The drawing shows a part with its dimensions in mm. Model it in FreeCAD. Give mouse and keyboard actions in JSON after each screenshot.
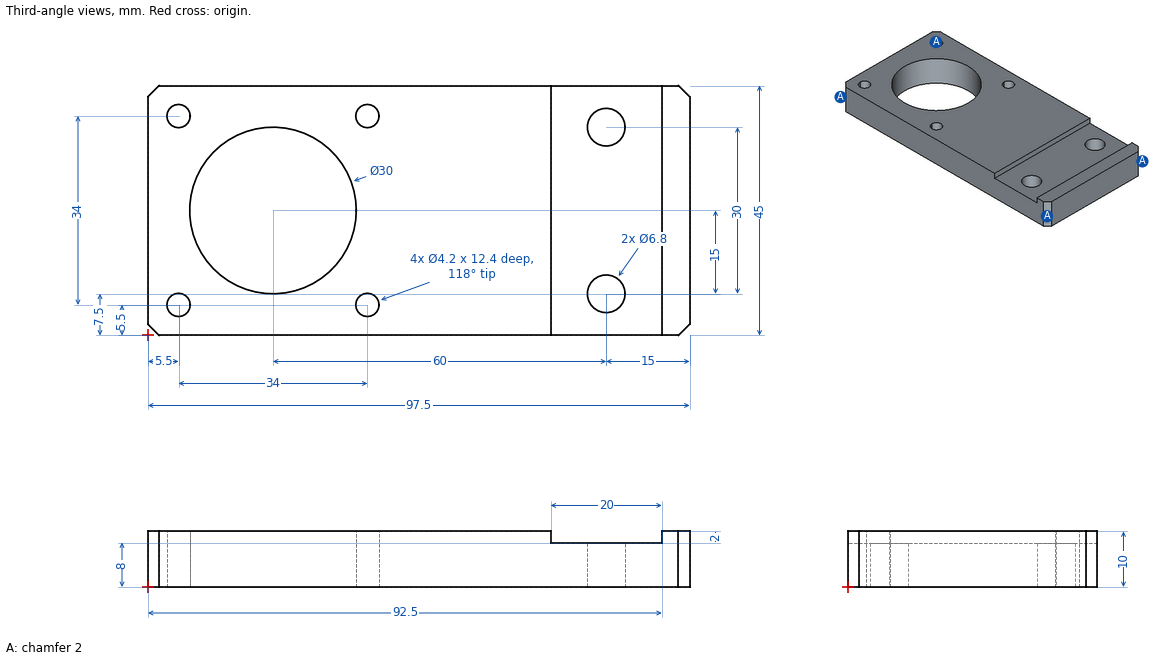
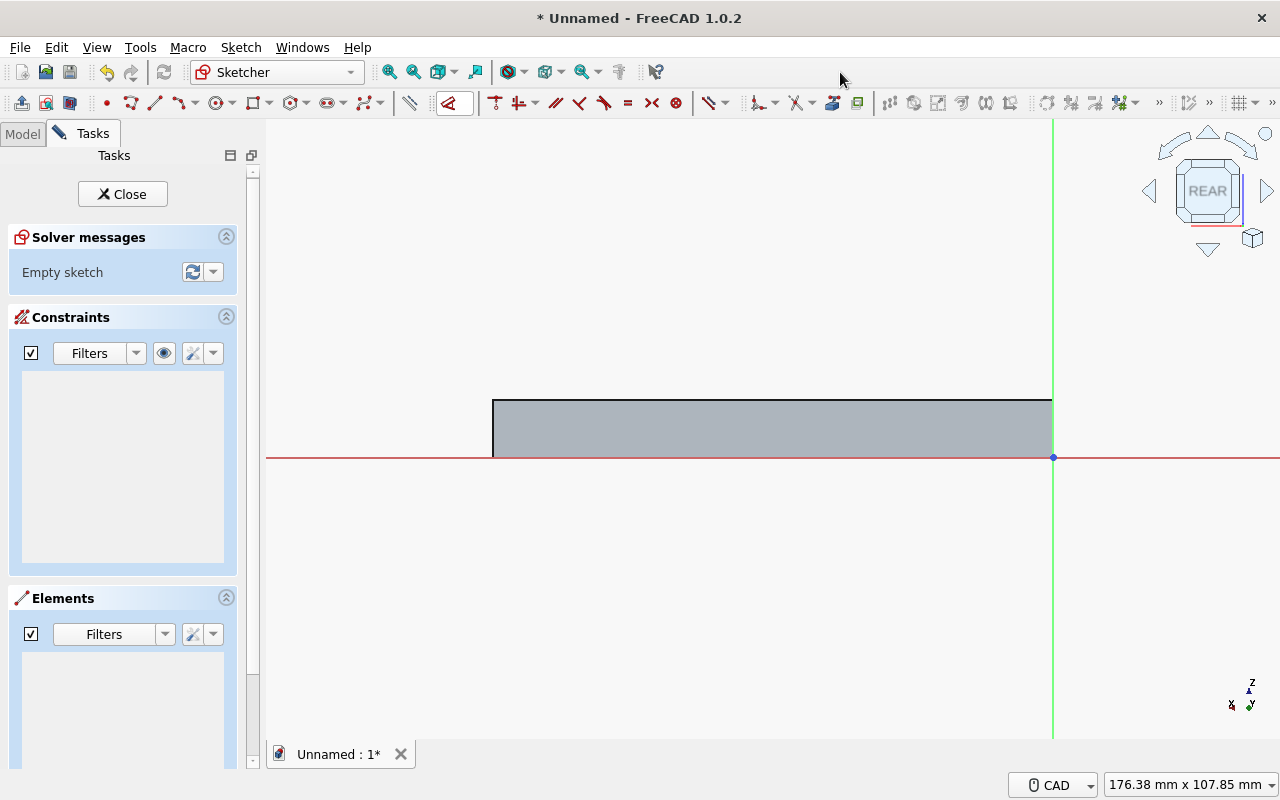
{"action": "scroll", "coordinate": [547, 400], "scroll_direction": "up", "scroll_amount": 8}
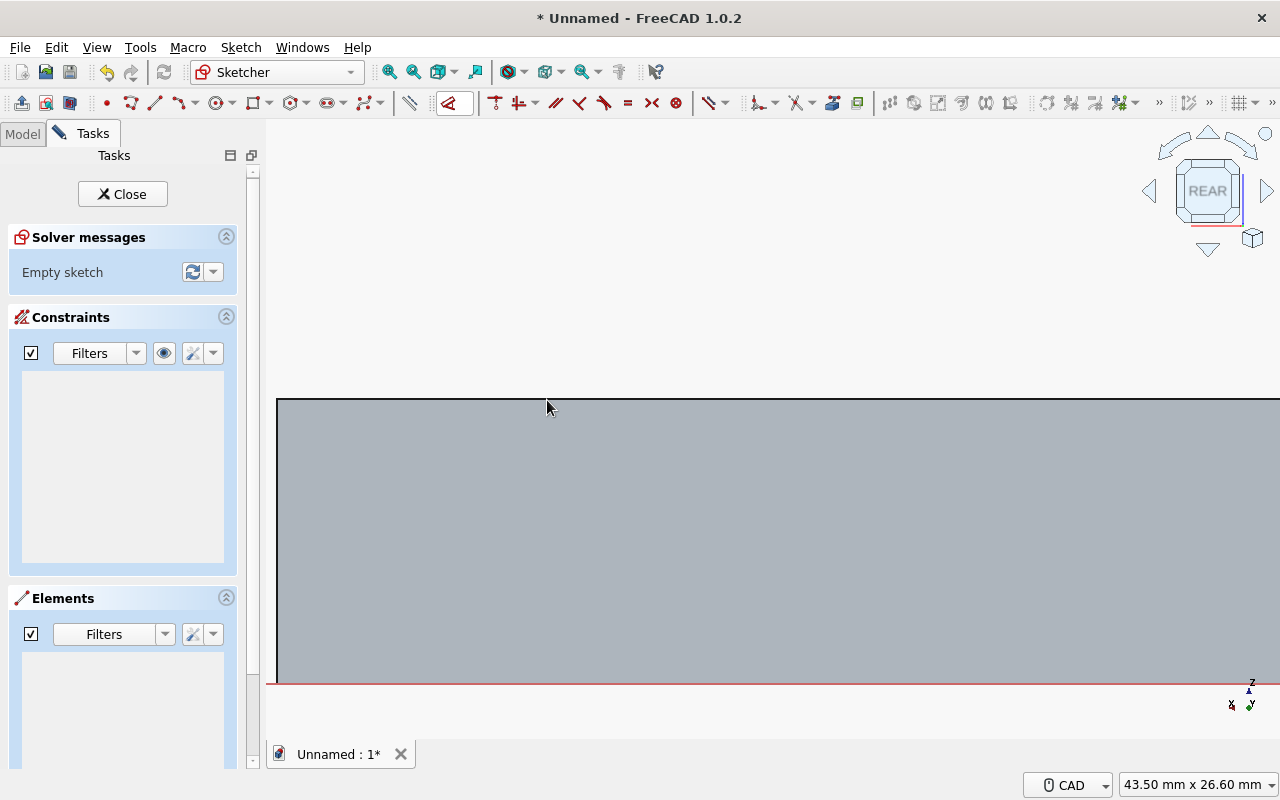
{"action": "left_click", "coordinate": [254, 104]}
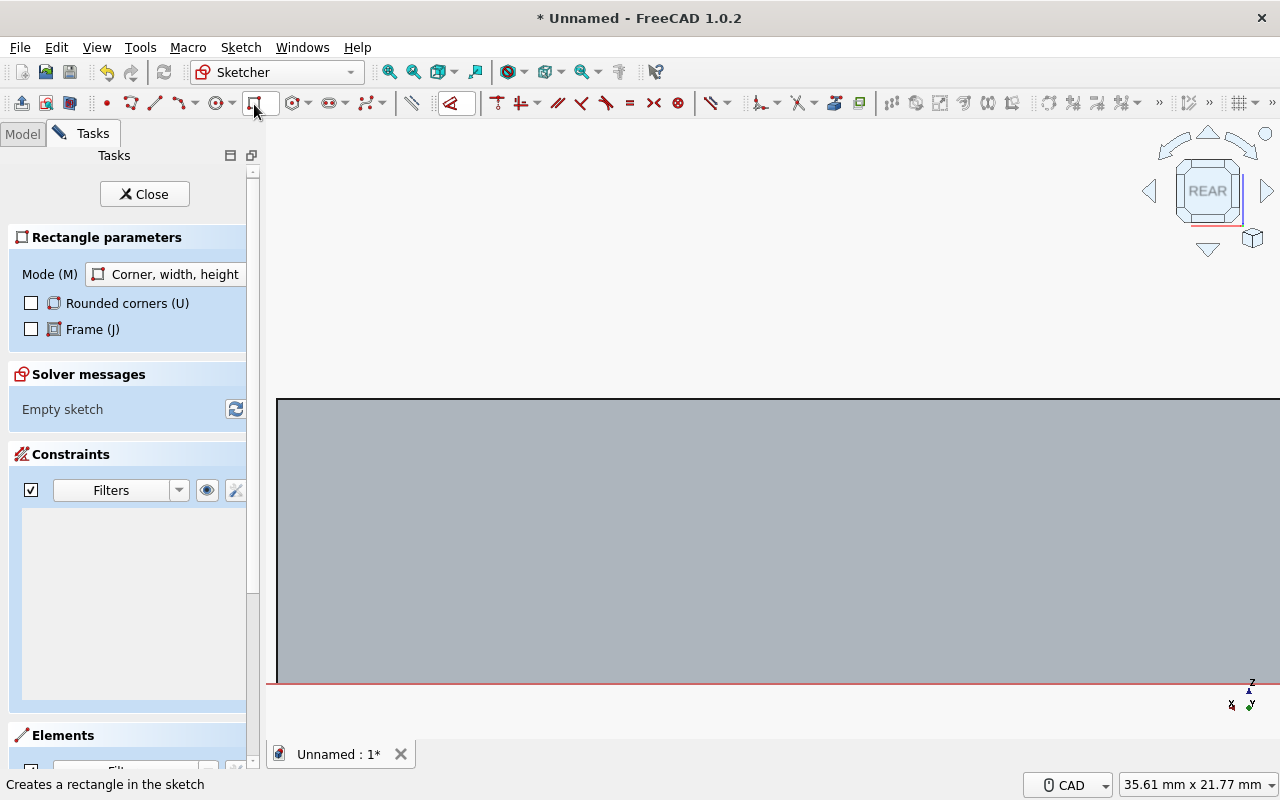
{"action": "left_click", "coordinate": [420, 399]}
{"action": "left_click", "coordinate": [989, 456]}
{"action": "key", "text": "Escape"}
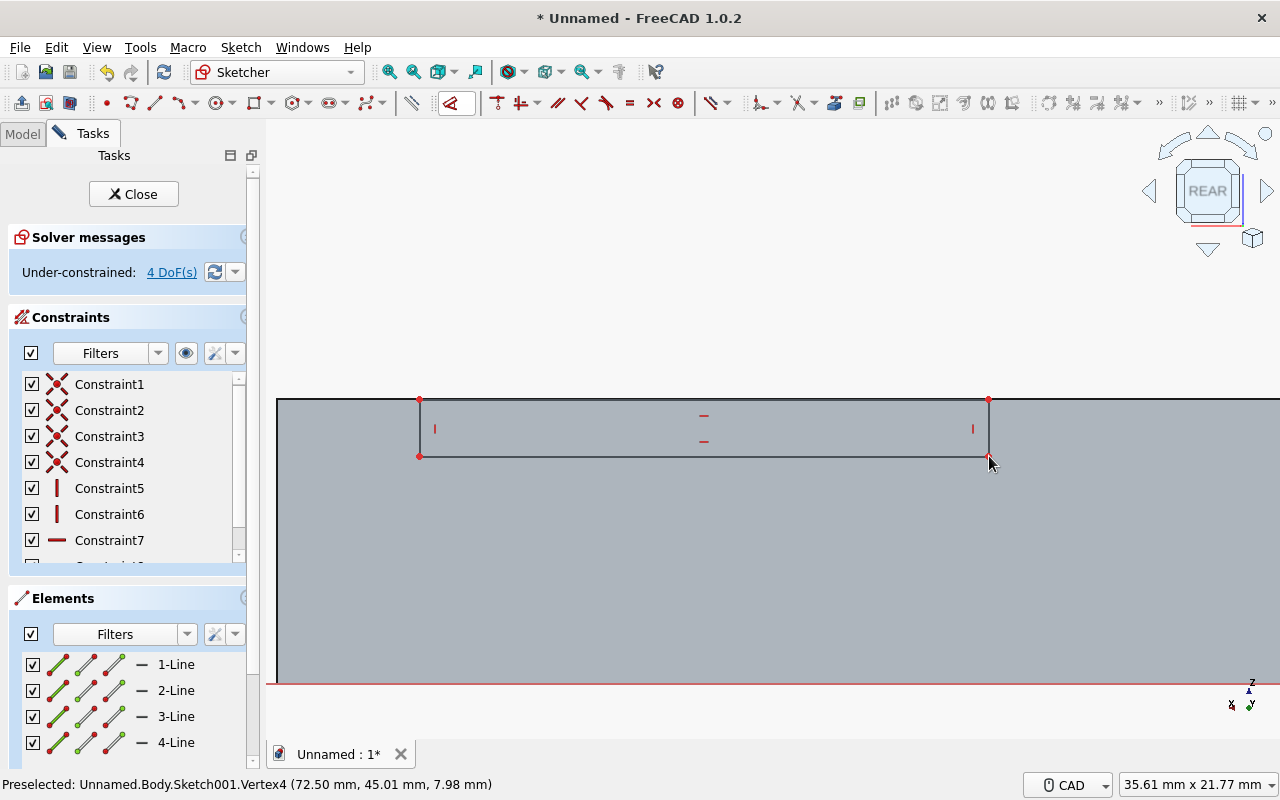
{"action": "left_click", "coordinate": [420, 417]}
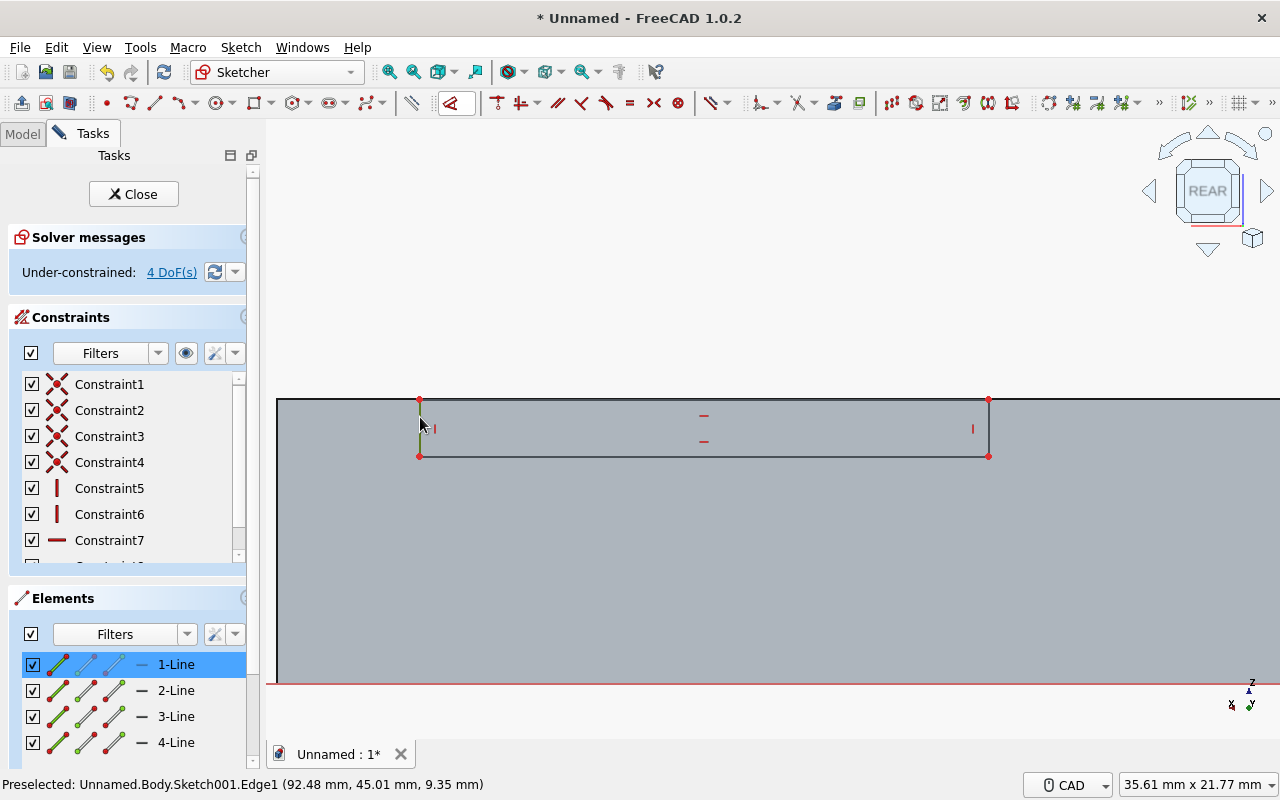
{"action": "key", "text": "i"}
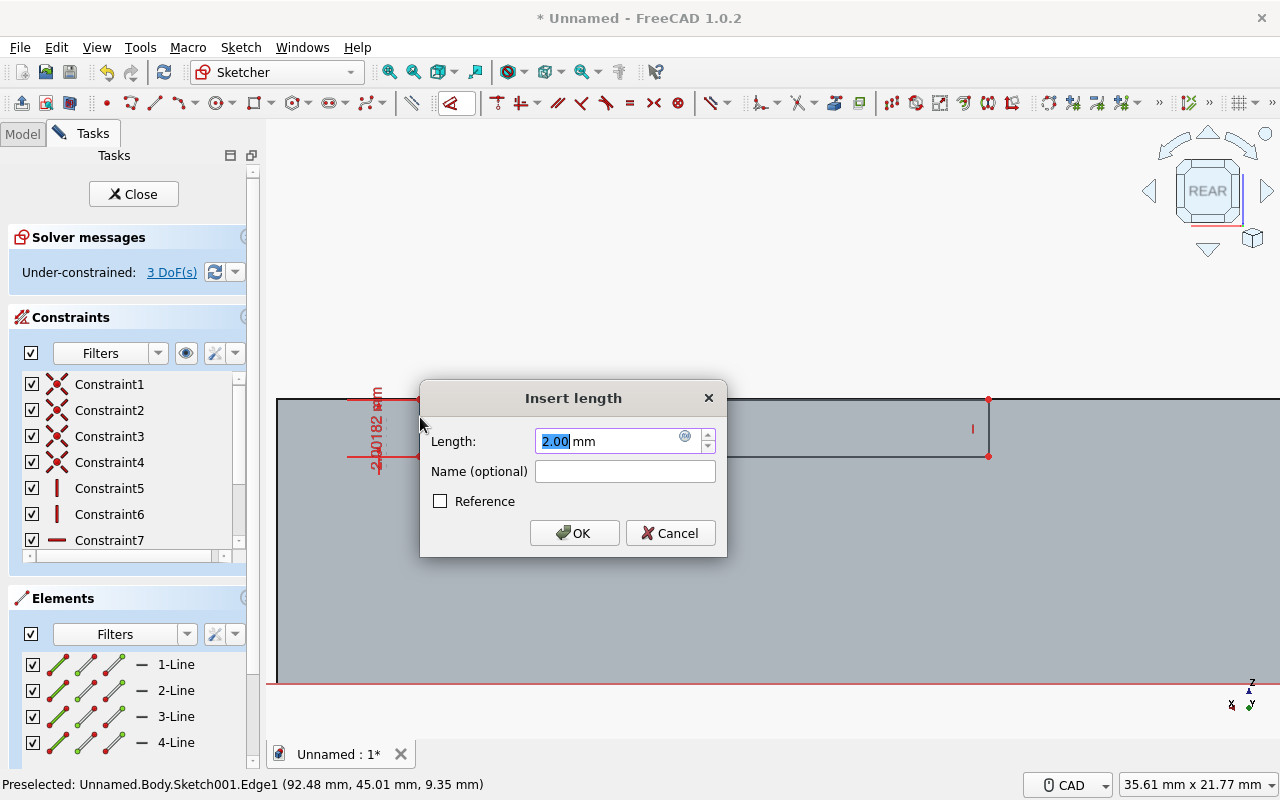
{"action": "type", "text": "2"}
{"action": "key", "text": "Return"}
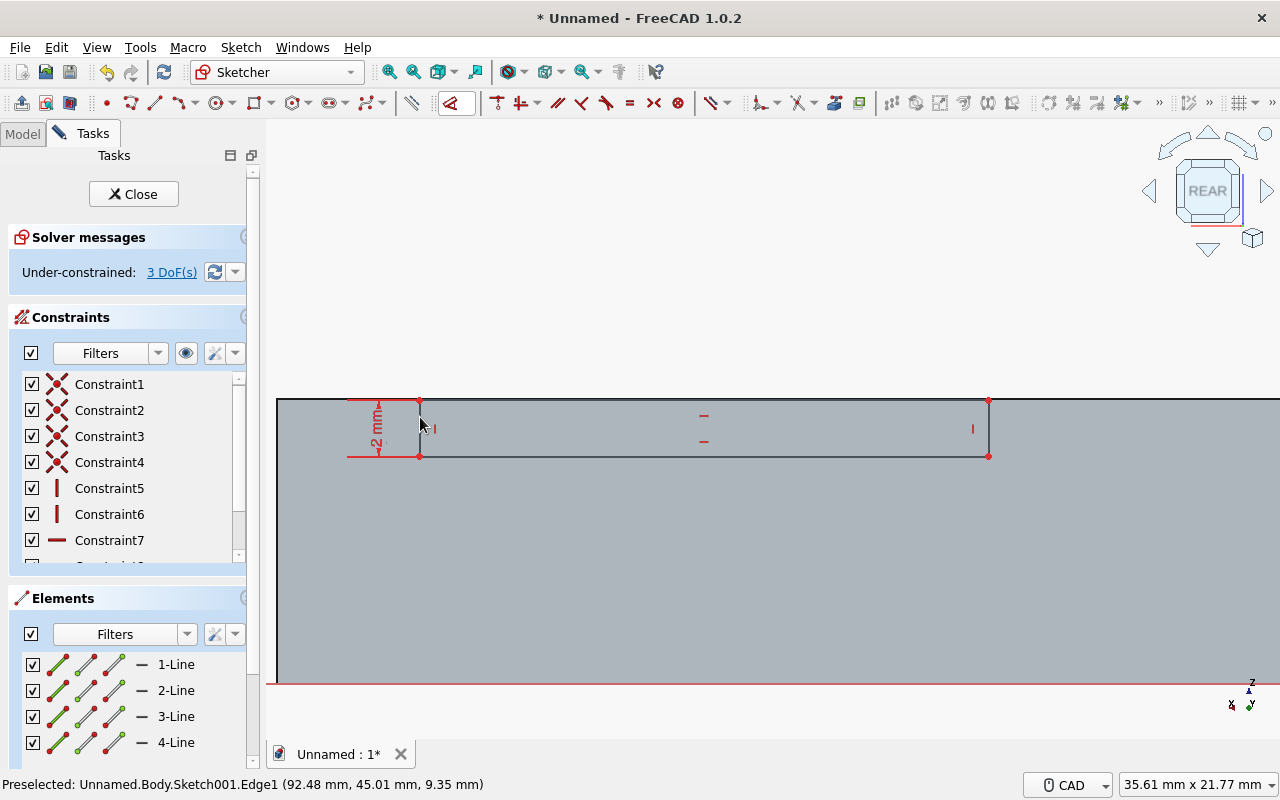
{"action": "left_click", "coordinate": [591, 457]}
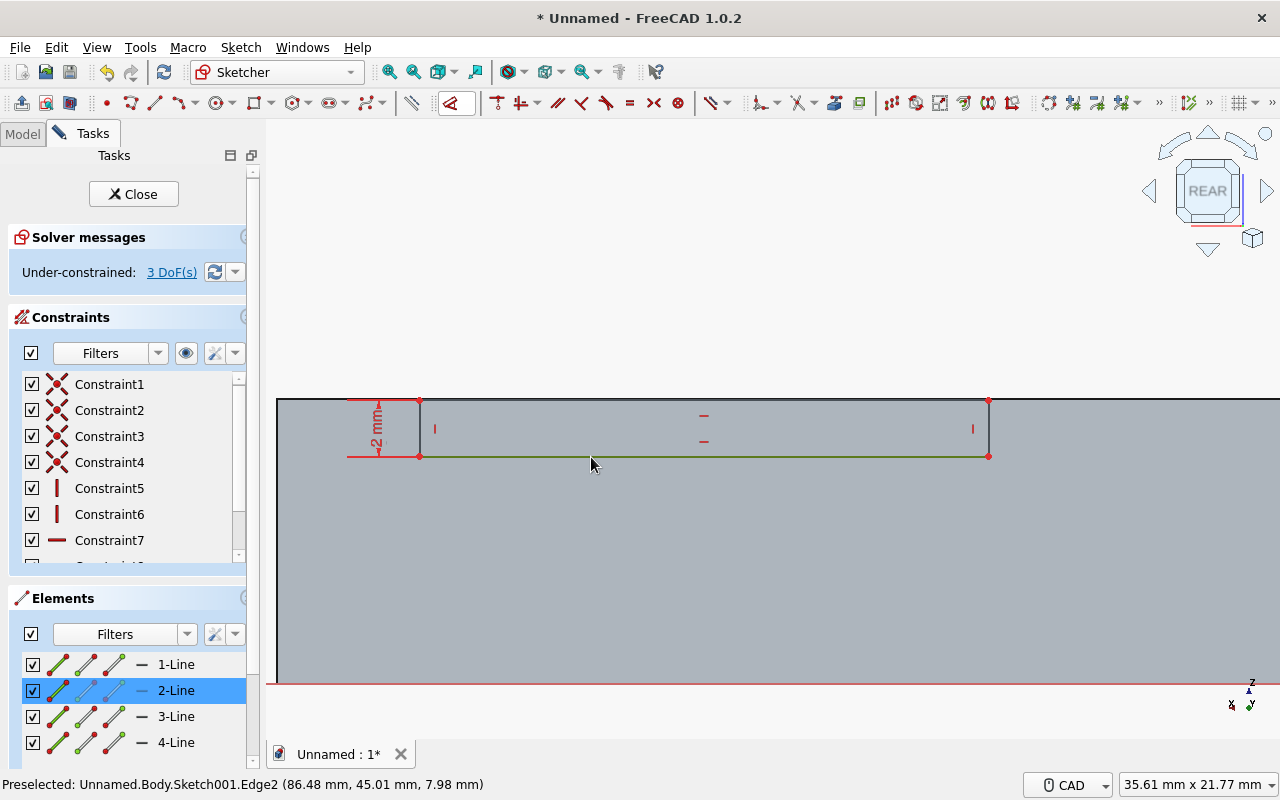
{"action": "key", "text": "l"}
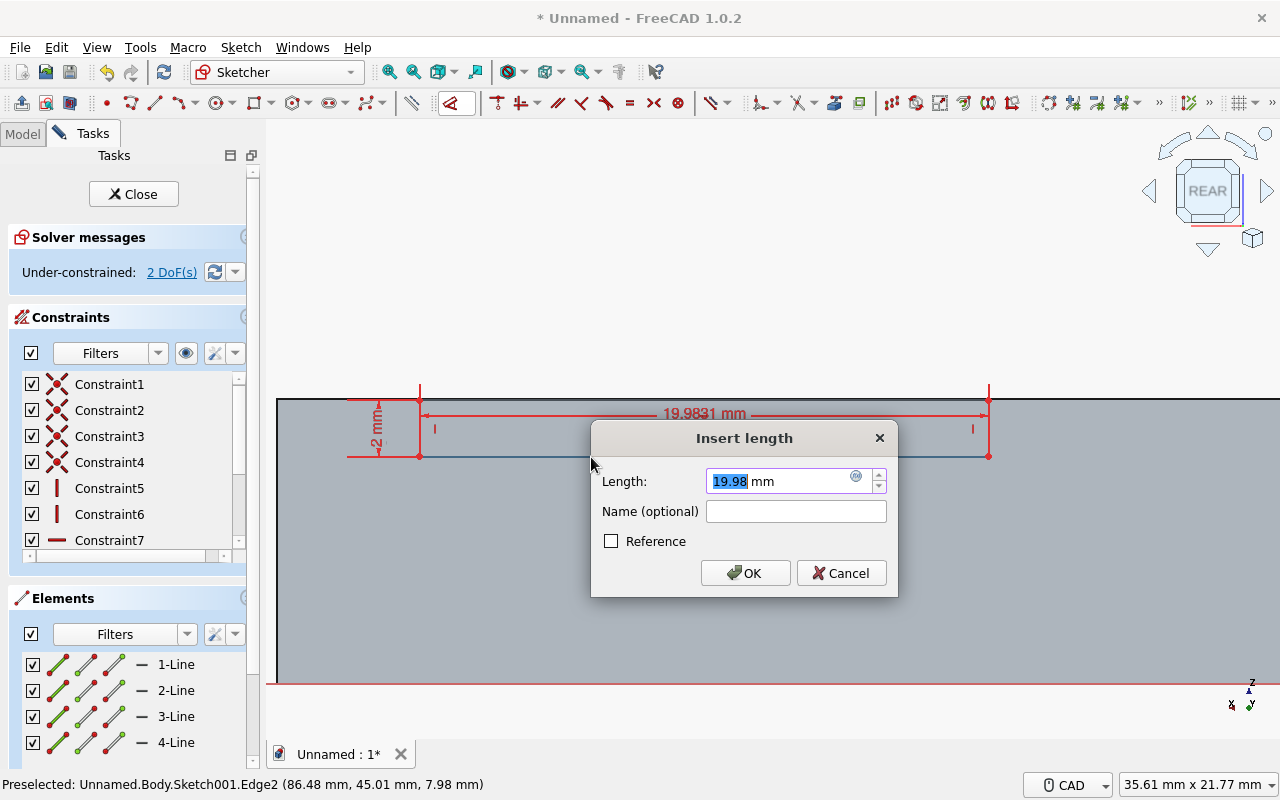
{"action": "type", "text": "20"}
{"action": "key", "text": "Return"}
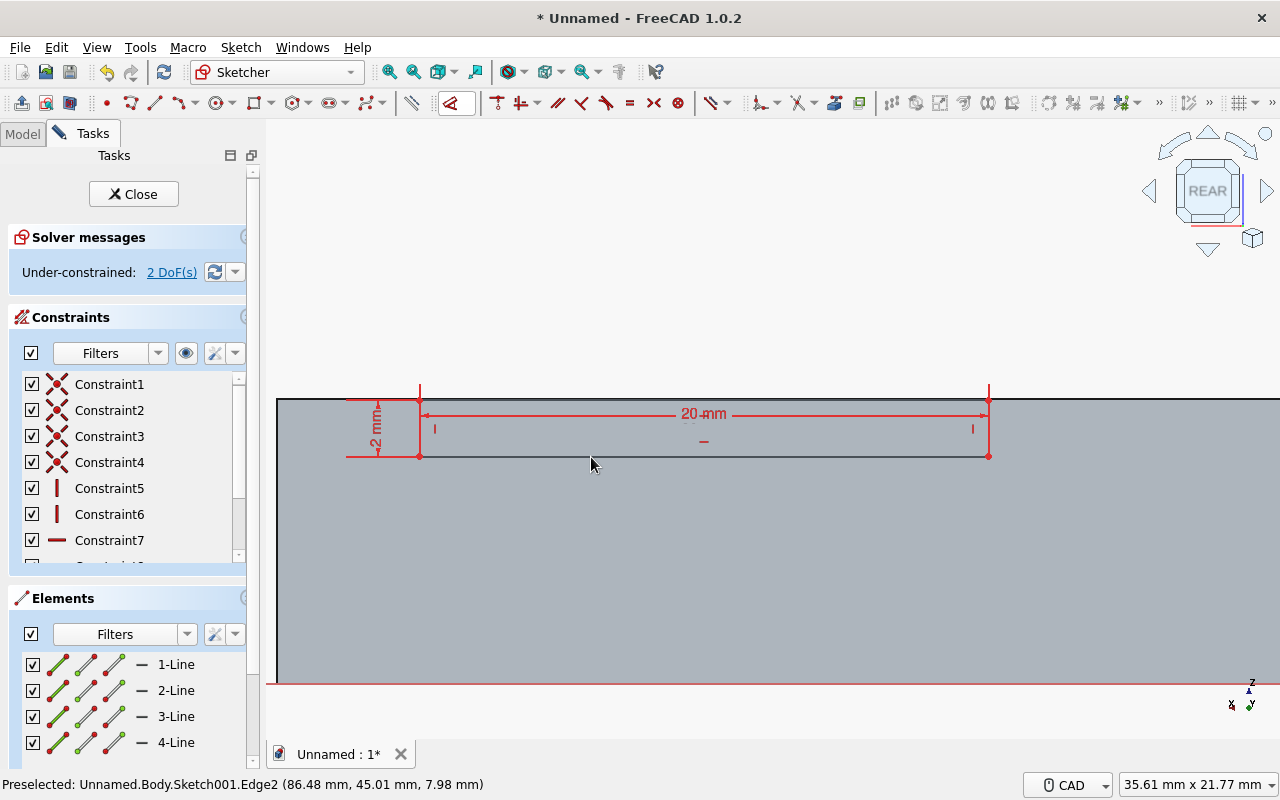
{"action": "left_click", "coordinate": [420, 457]}